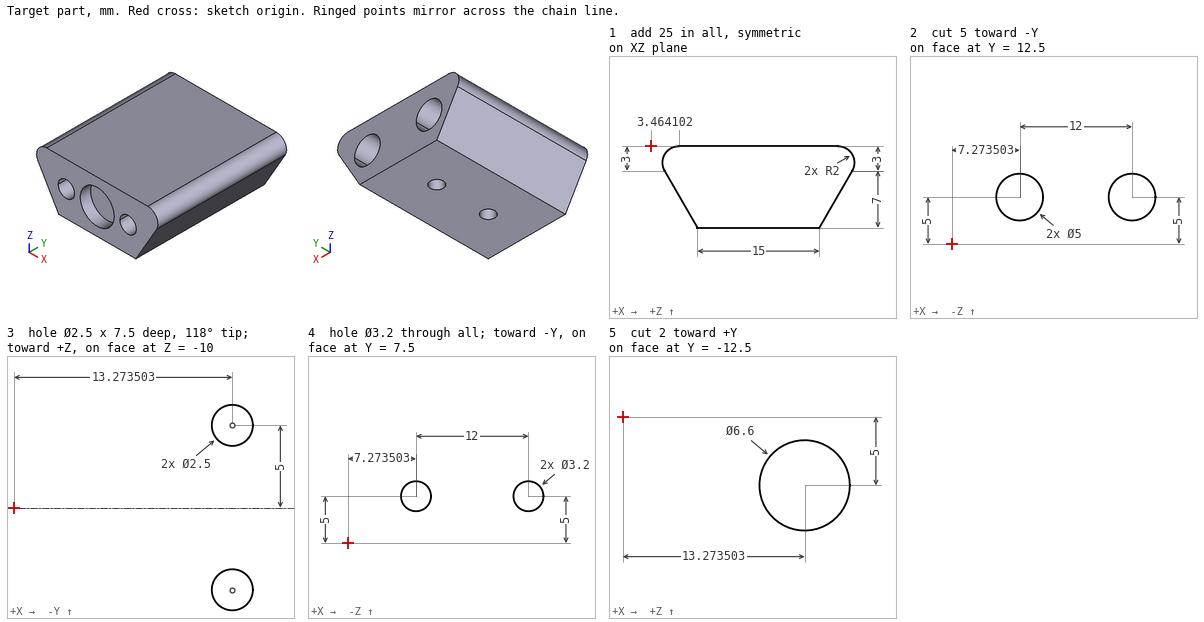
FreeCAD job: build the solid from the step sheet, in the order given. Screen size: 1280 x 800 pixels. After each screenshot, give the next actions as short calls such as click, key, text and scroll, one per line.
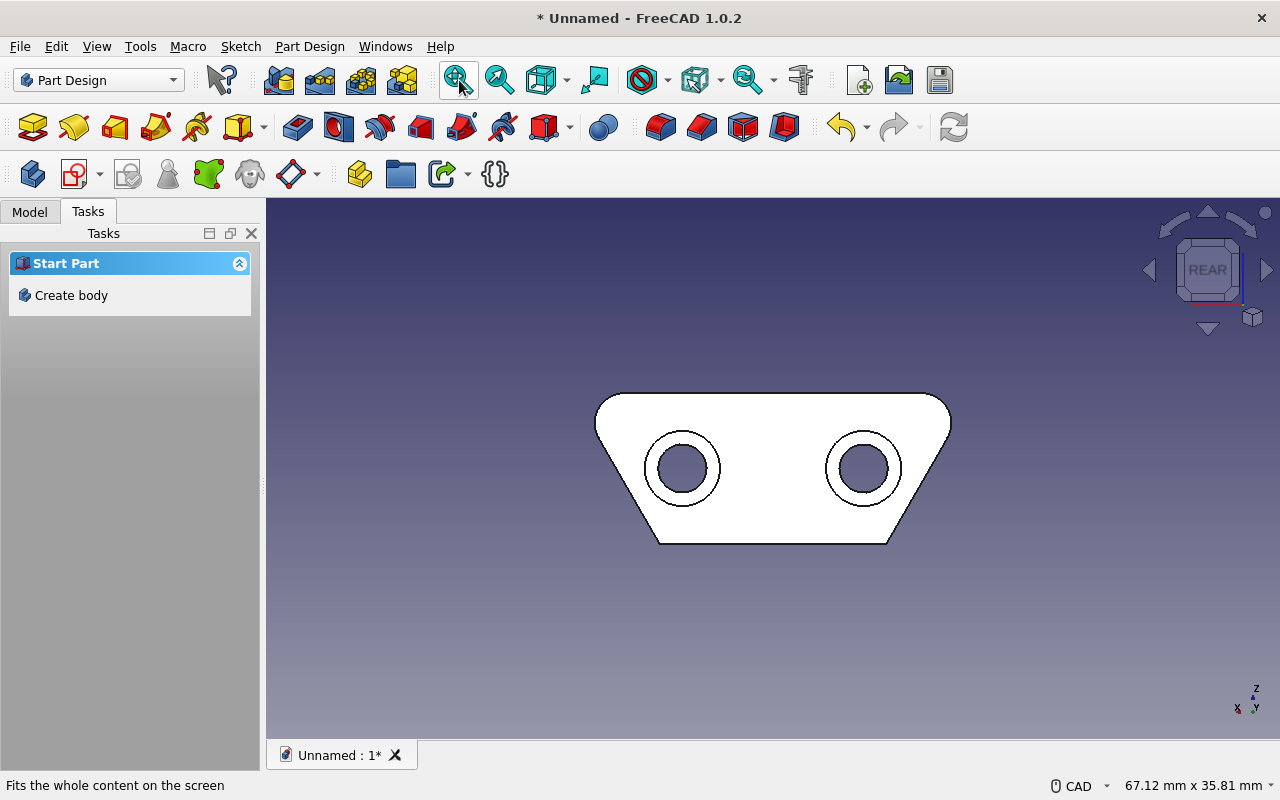
key(0)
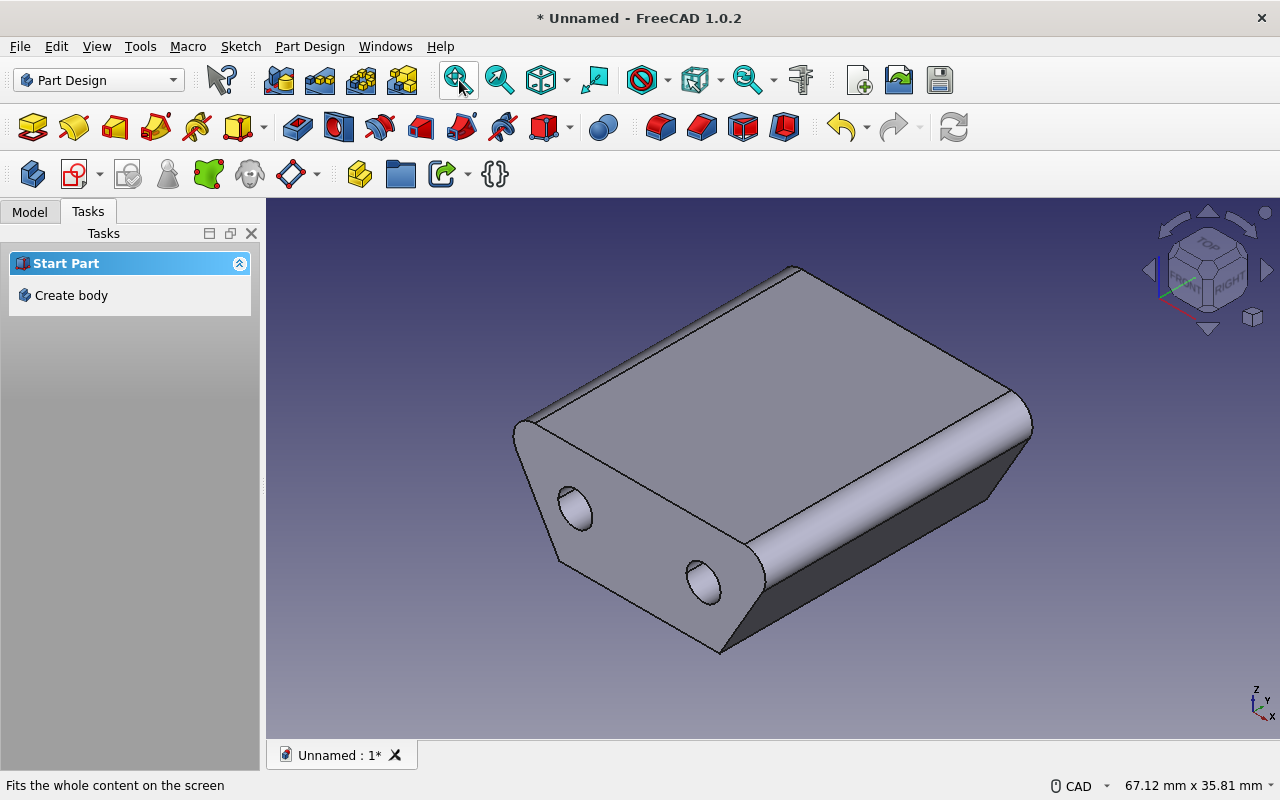
click(639, 545)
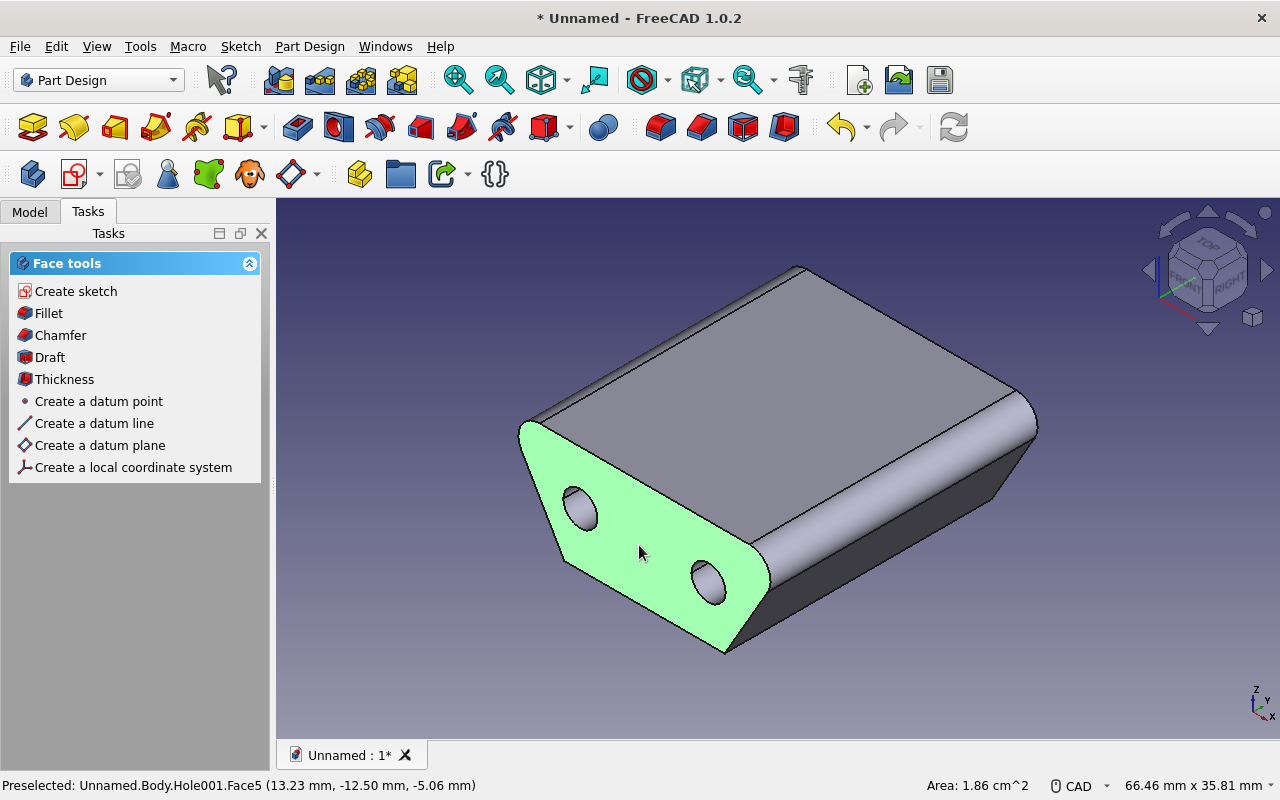
click(74, 174)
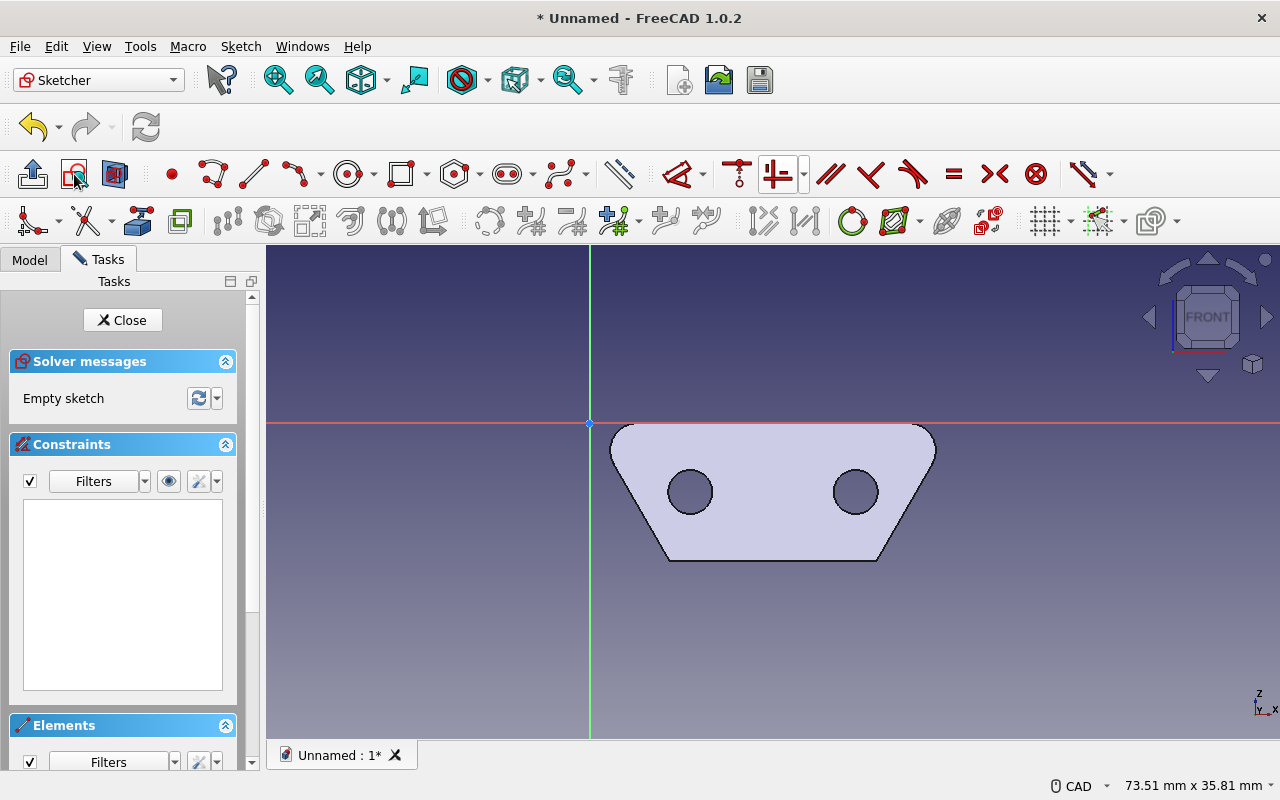
scroll(803, 492, up, 6)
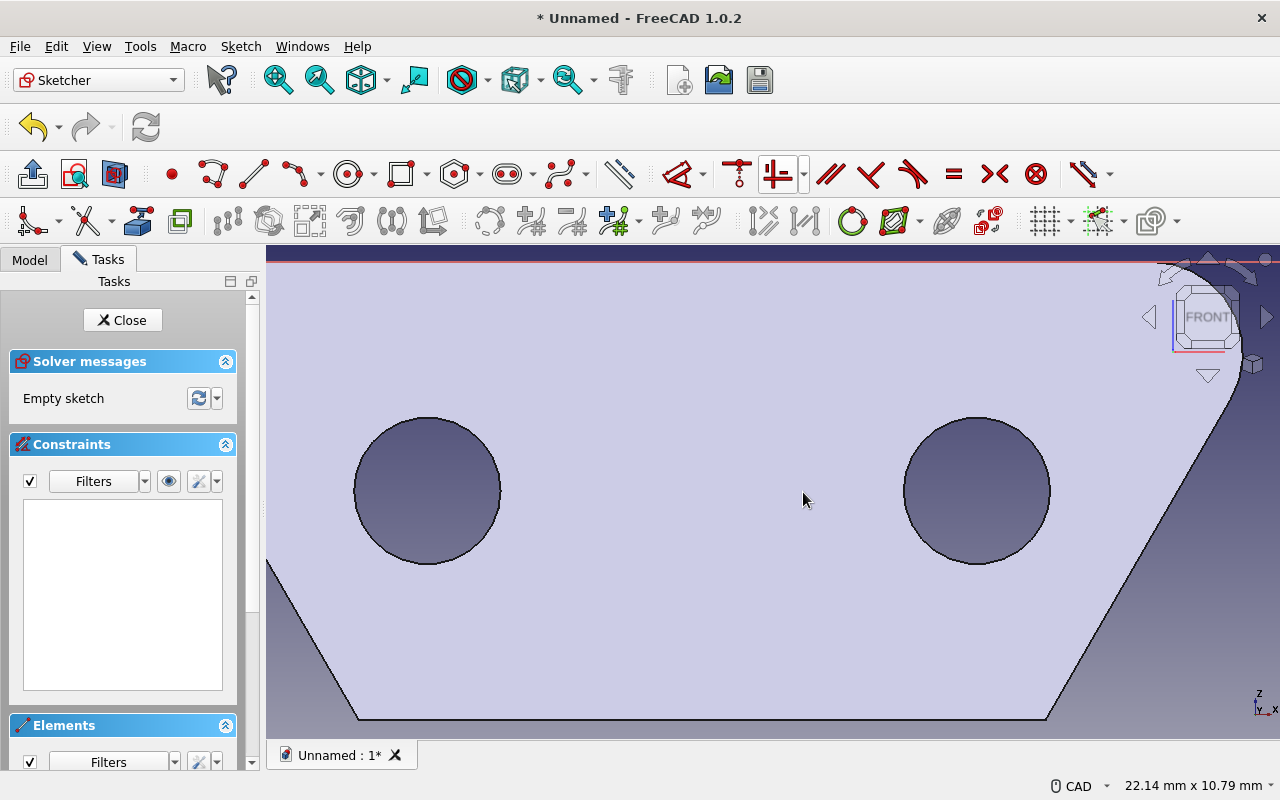
click(348, 174)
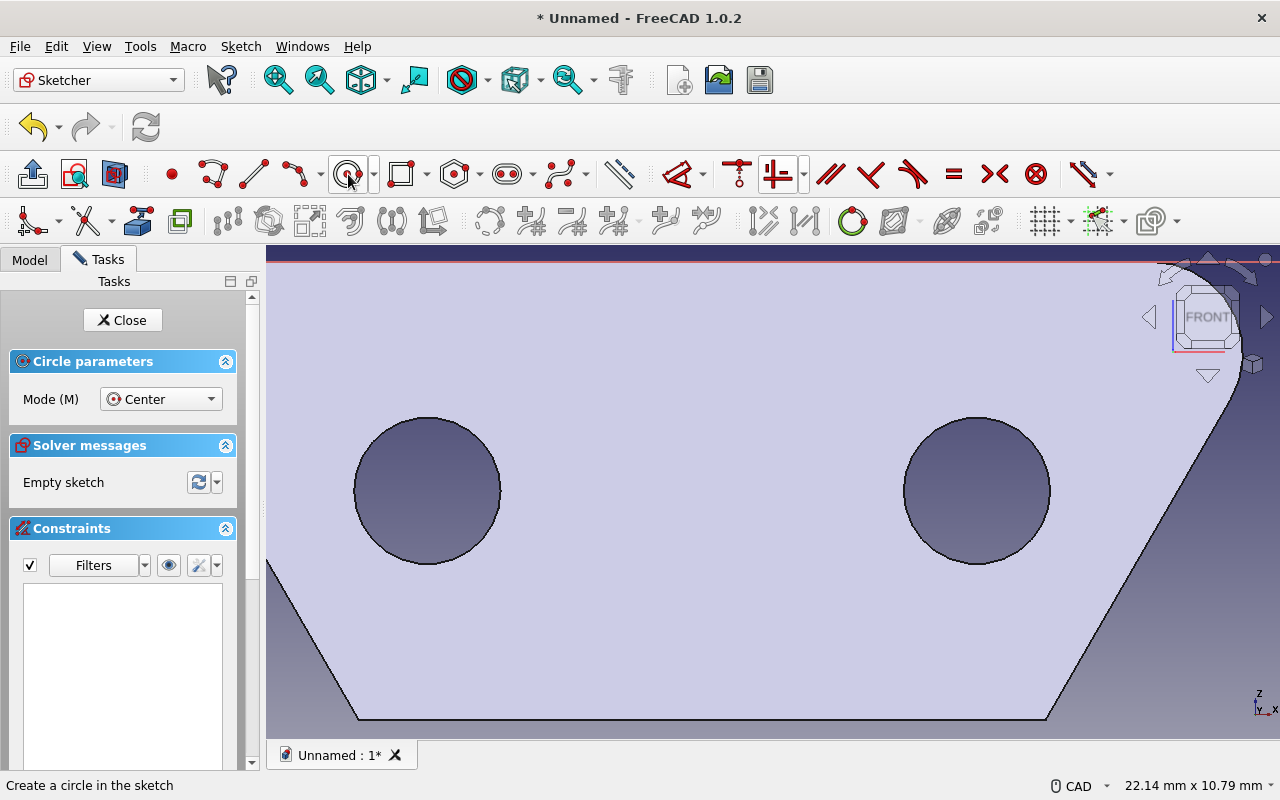
click(702, 491)
click(809, 384)
key(Escape)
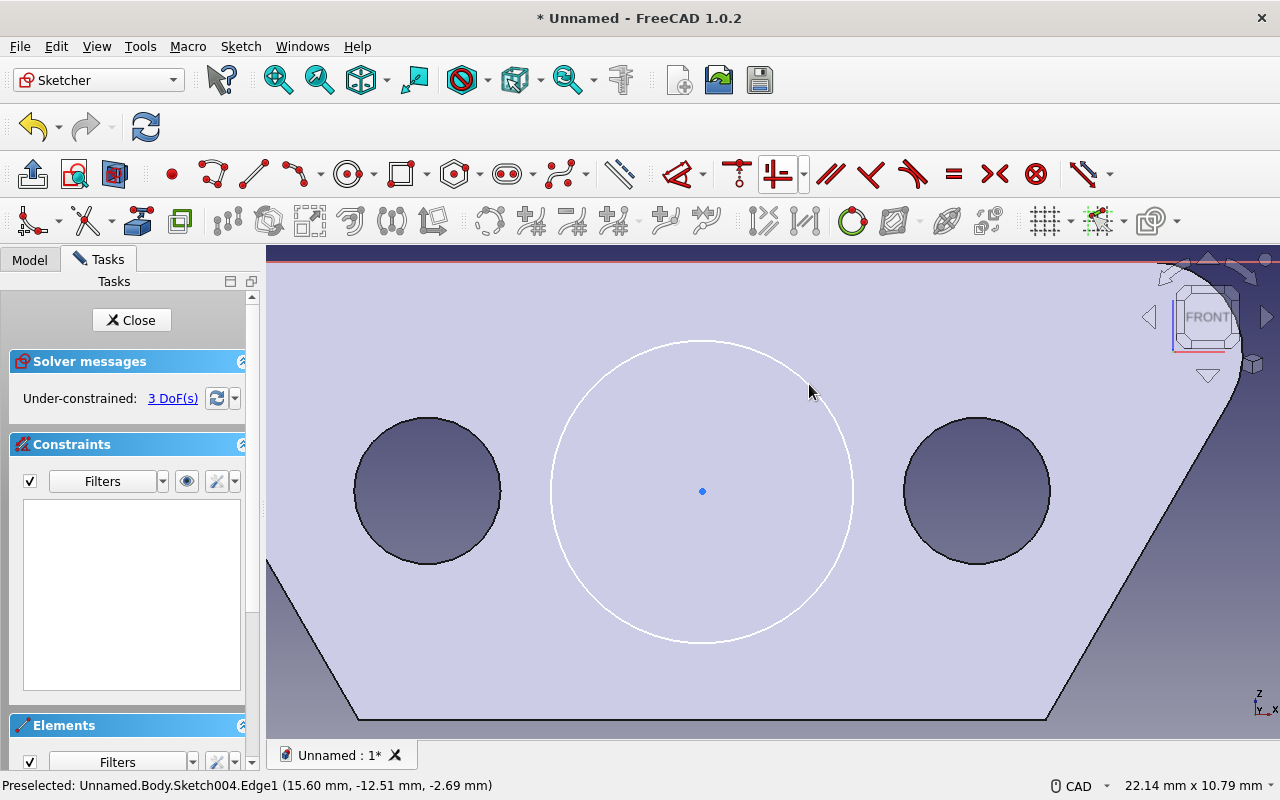
click(676, 174)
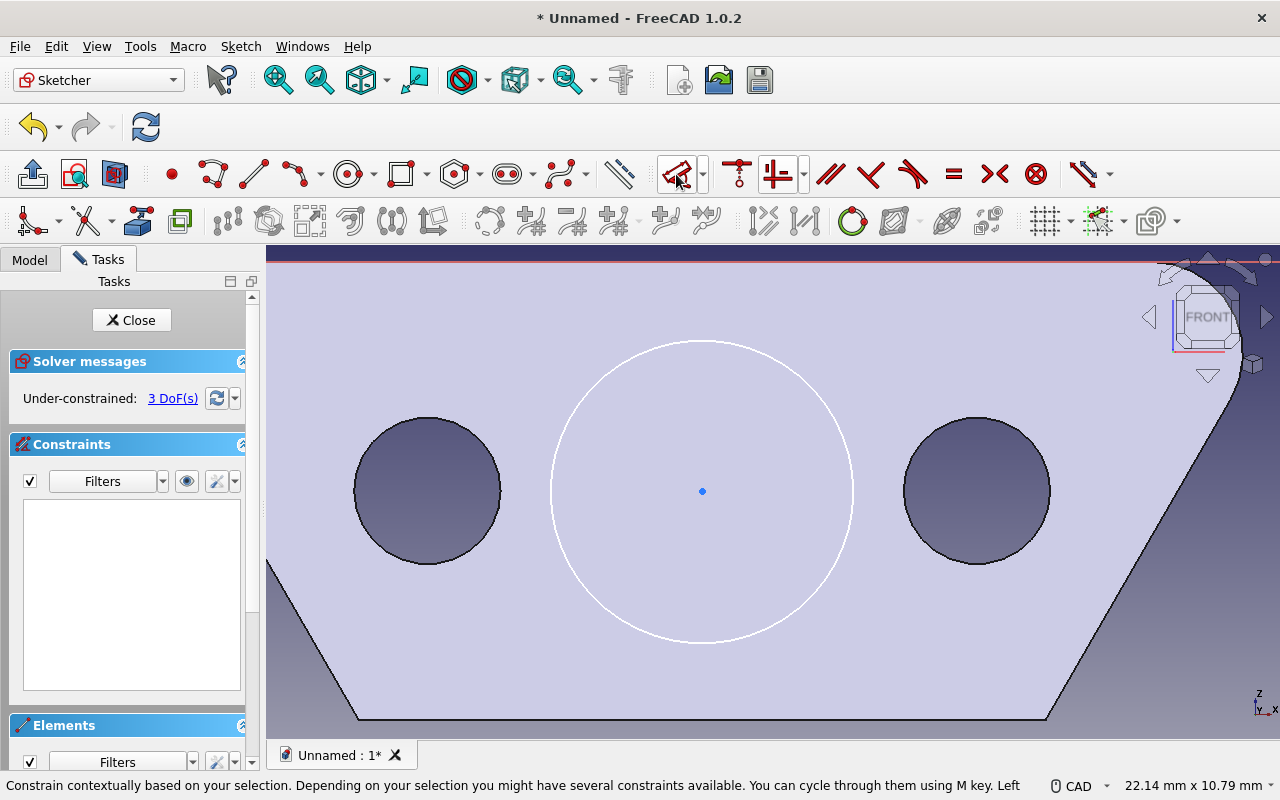
click(809, 385)
click(832, 362)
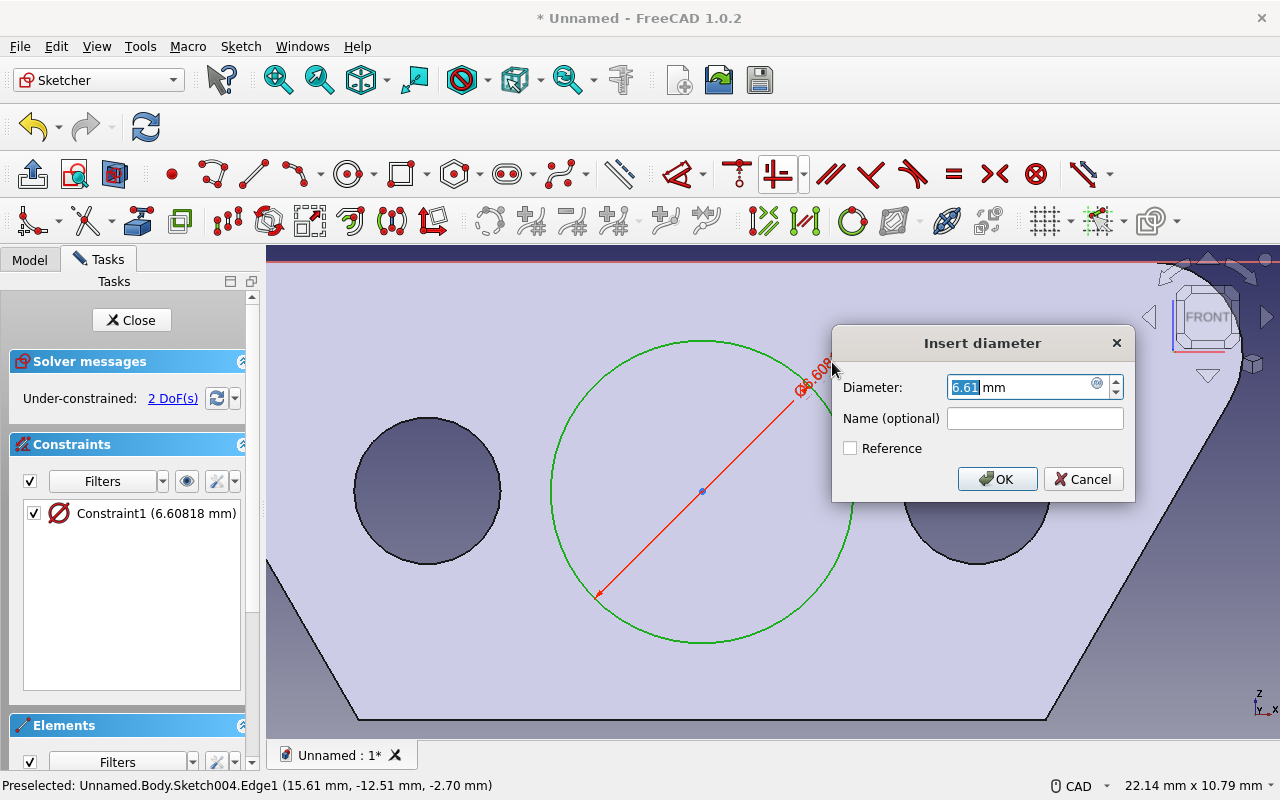
text(6.6)
key(Return)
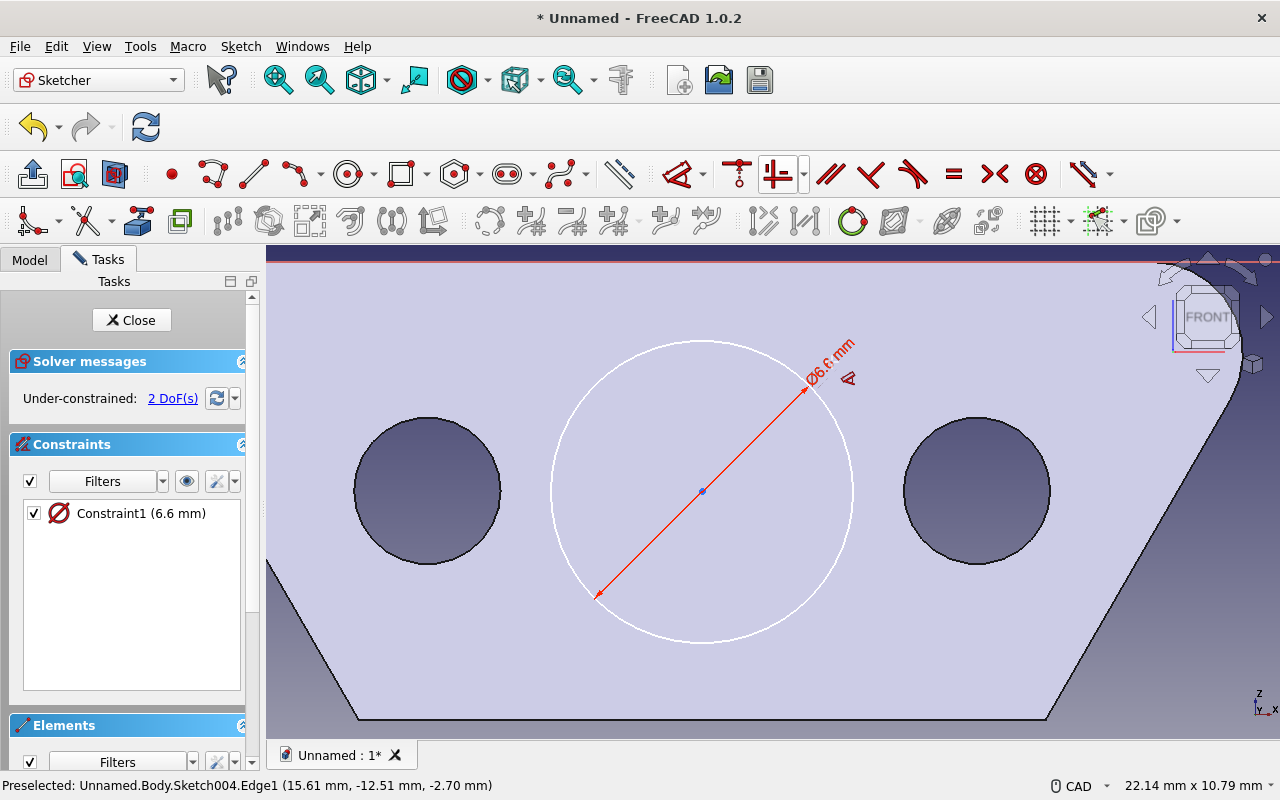
click(702, 492)
click(736, 383)